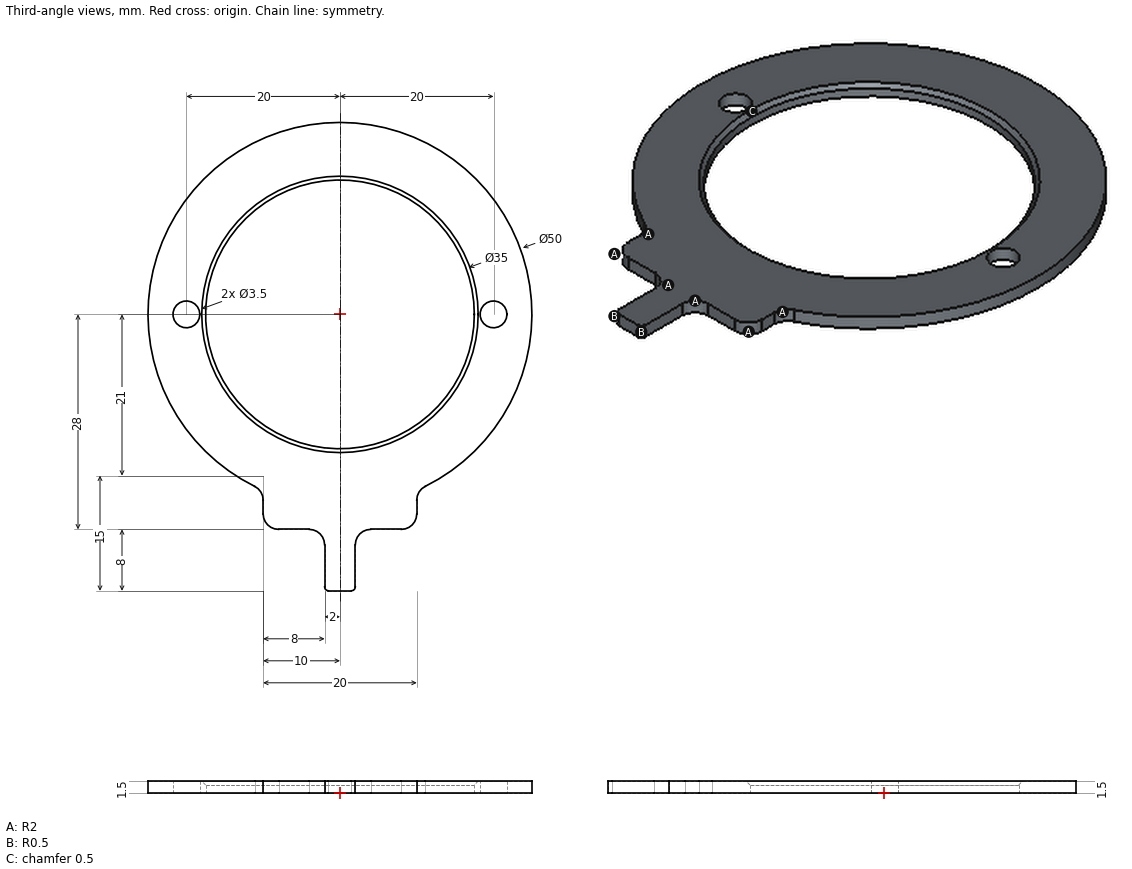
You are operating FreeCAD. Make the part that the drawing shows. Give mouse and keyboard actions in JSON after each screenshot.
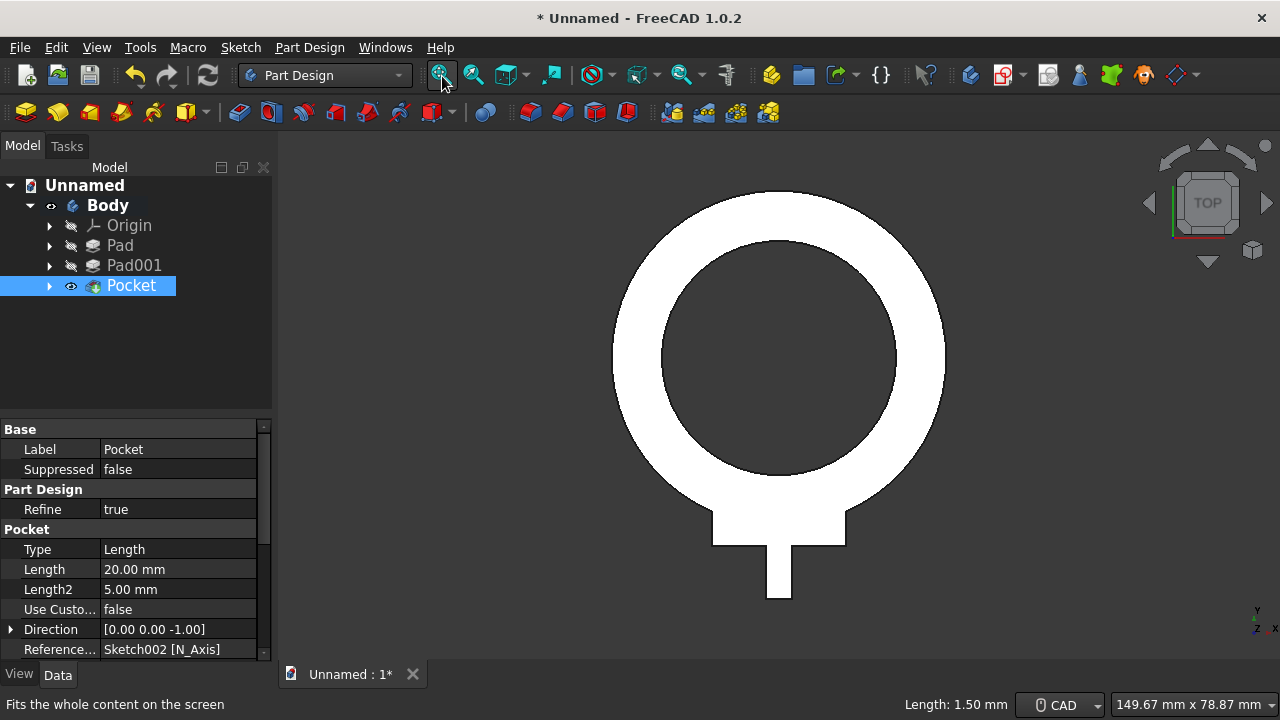
{"action": "scroll", "coordinate": [846, 511], "scroll_direction": "up", "scroll_amount": 7}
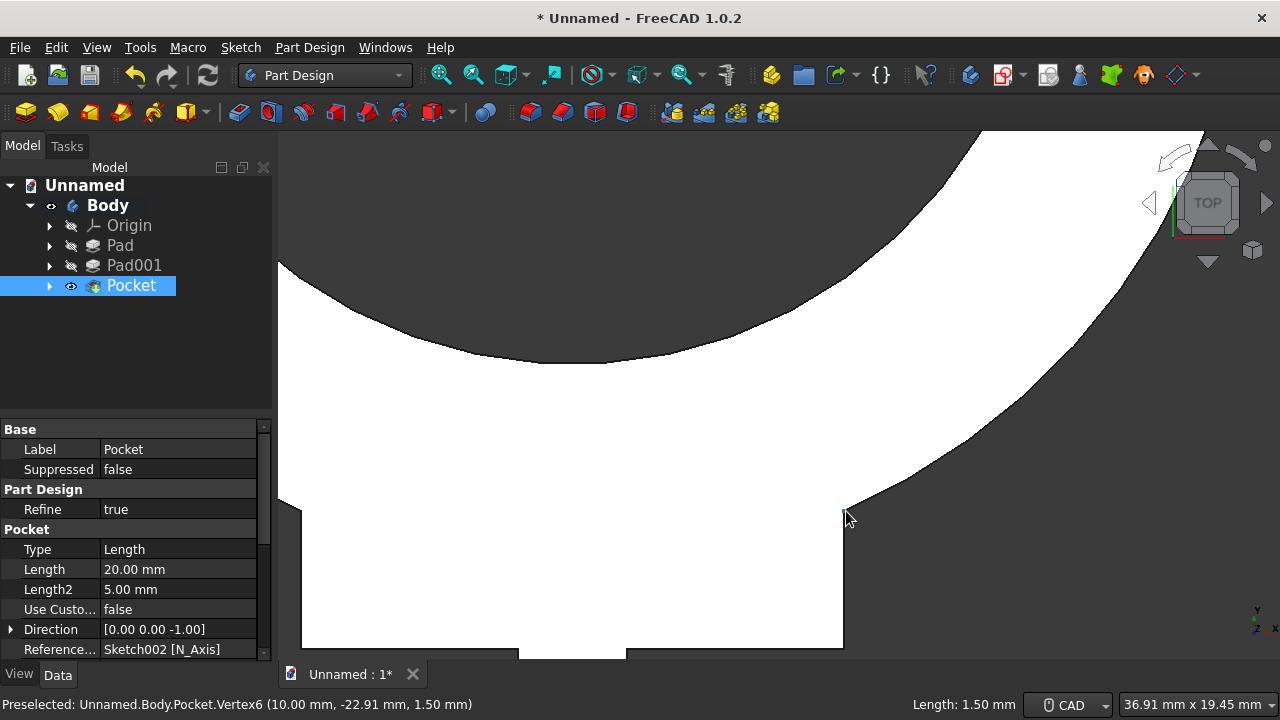
{"action": "left_click", "coordinate": [442, 76]}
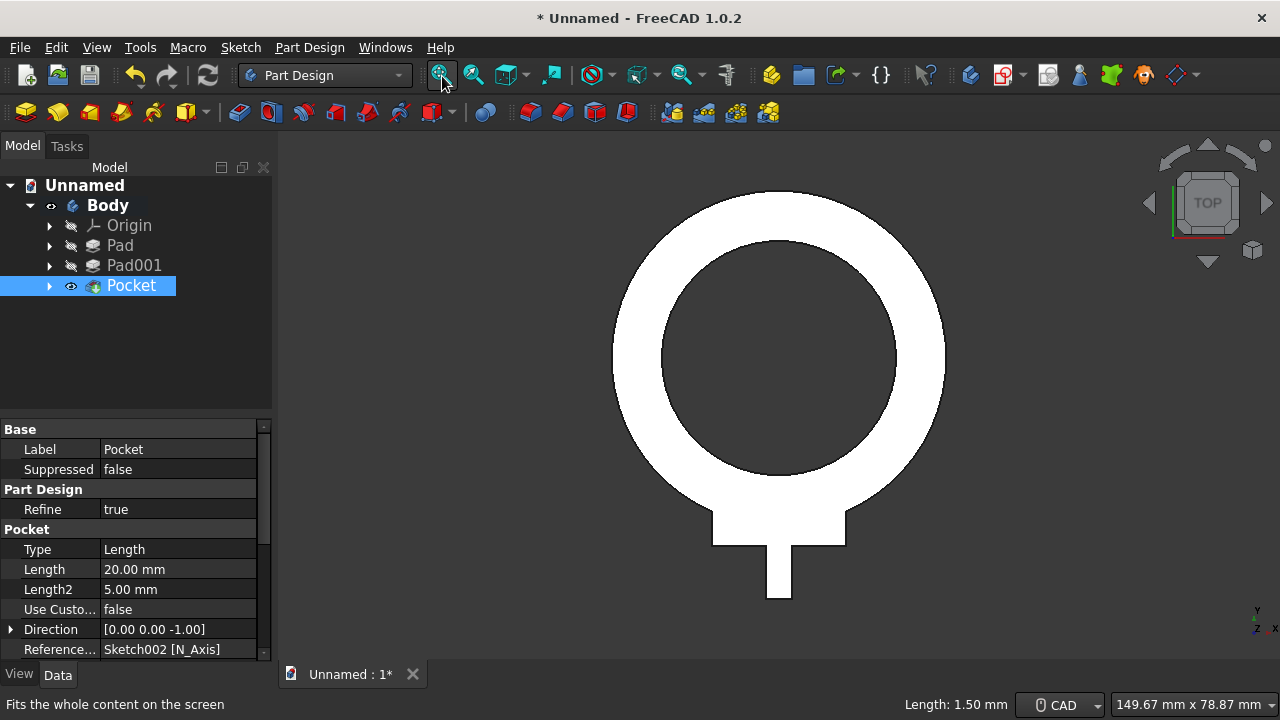
{"action": "key", "text": "1"}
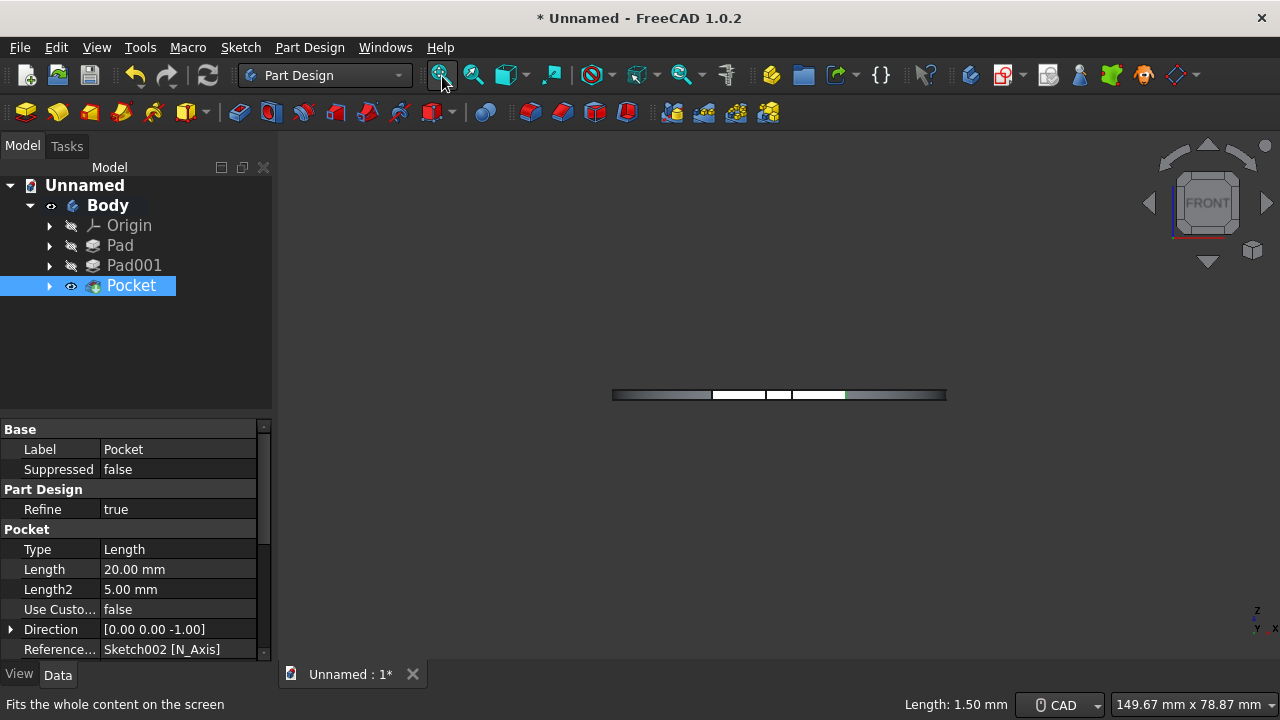
{"action": "left_click", "coordinate": [442, 76]}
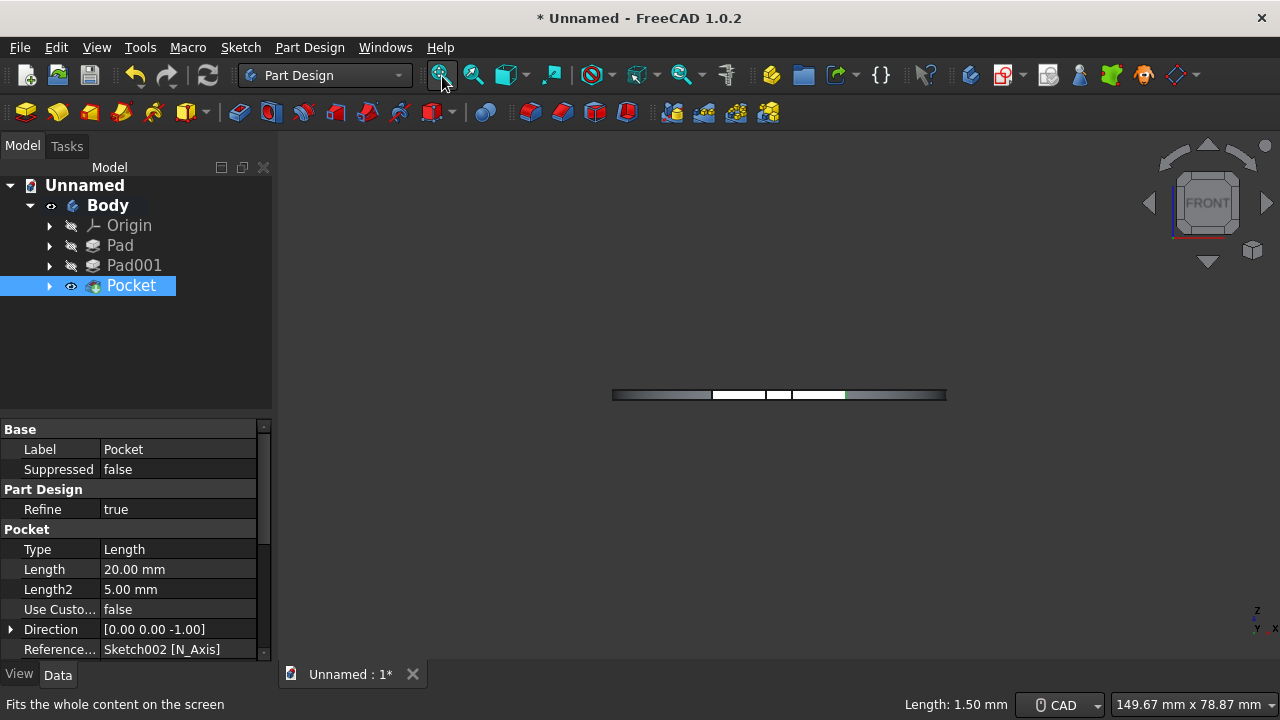
{"action": "scroll", "coordinate": [846, 394], "scroll_direction": "up", "scroll_amount": 7}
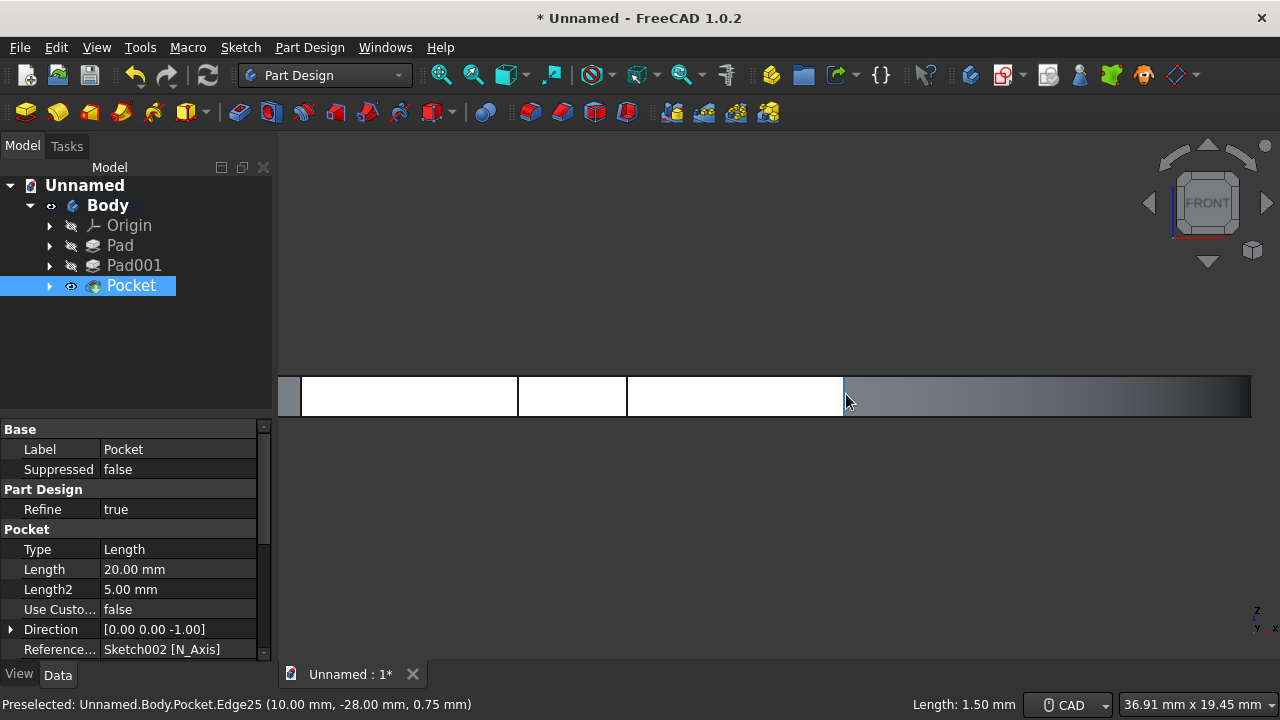
{"action": "left_click", "coordinate": [442, 76]}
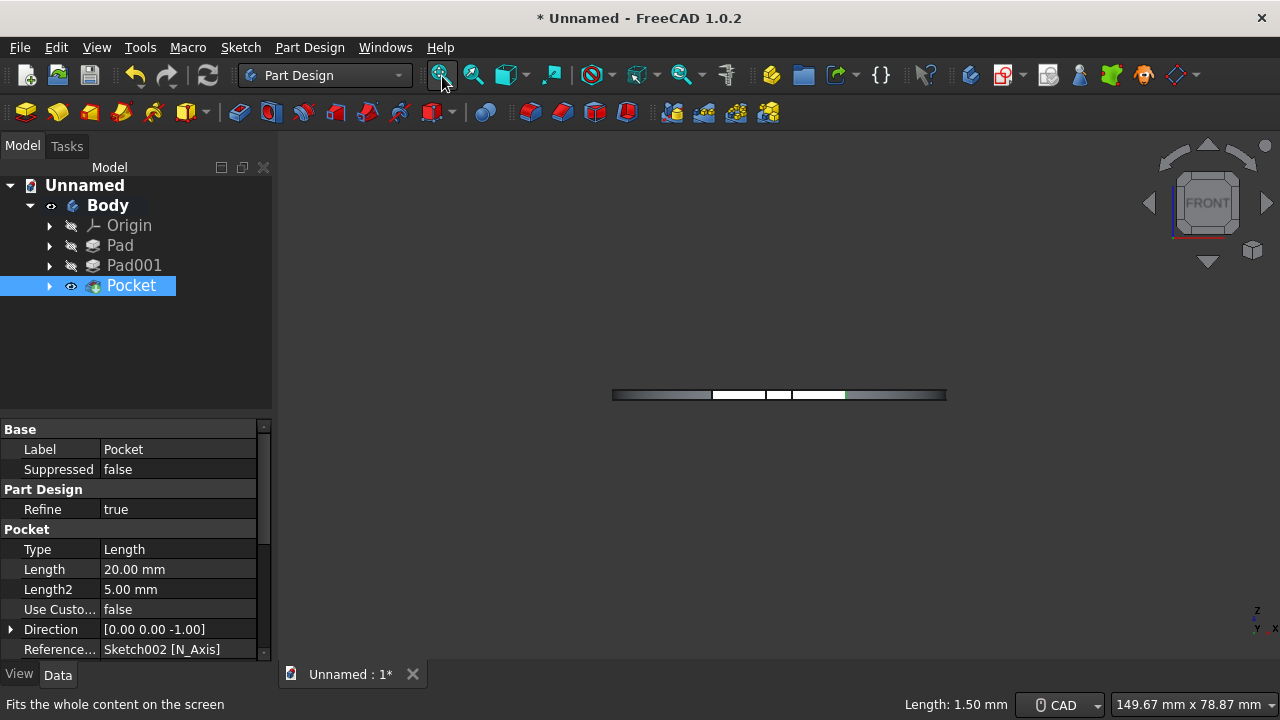
{"action": "key", "text": "3"}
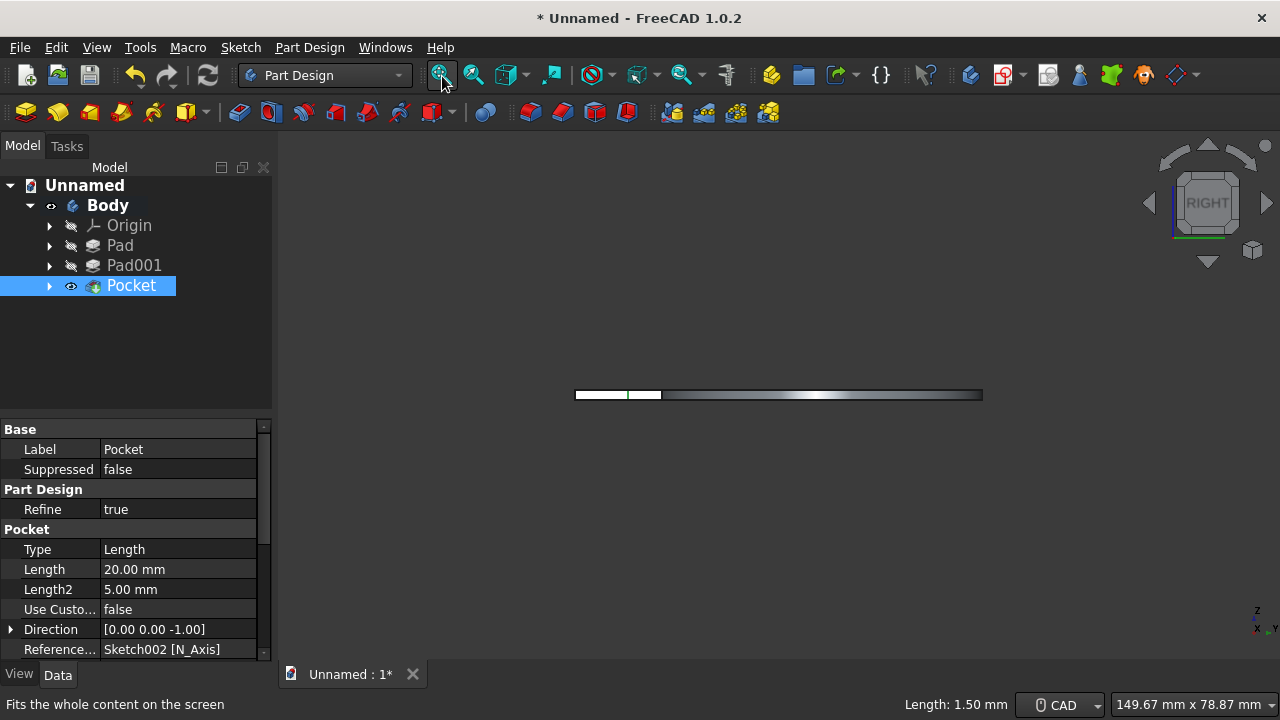
{"action": "left_click", "coordinate": [442, 76]}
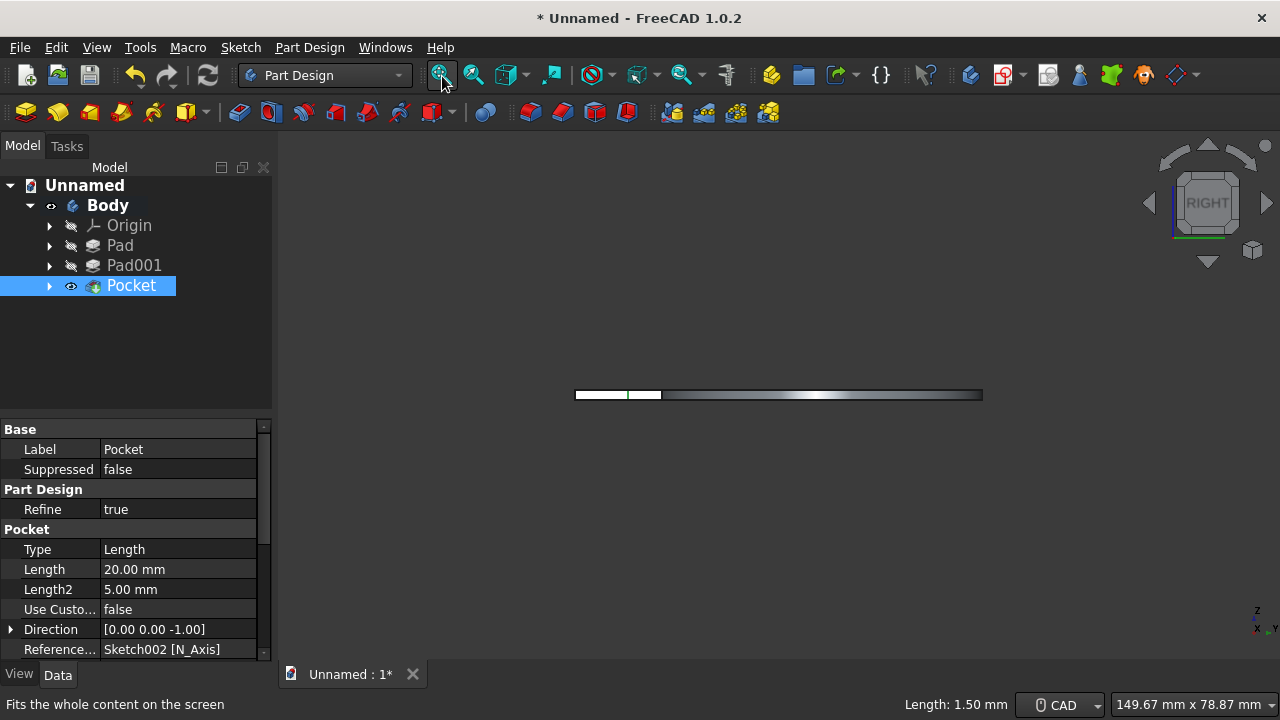
{"action": "scroll", "coordinate": [662, 394], "scroll_direction": "up", "scroll_amount": 7}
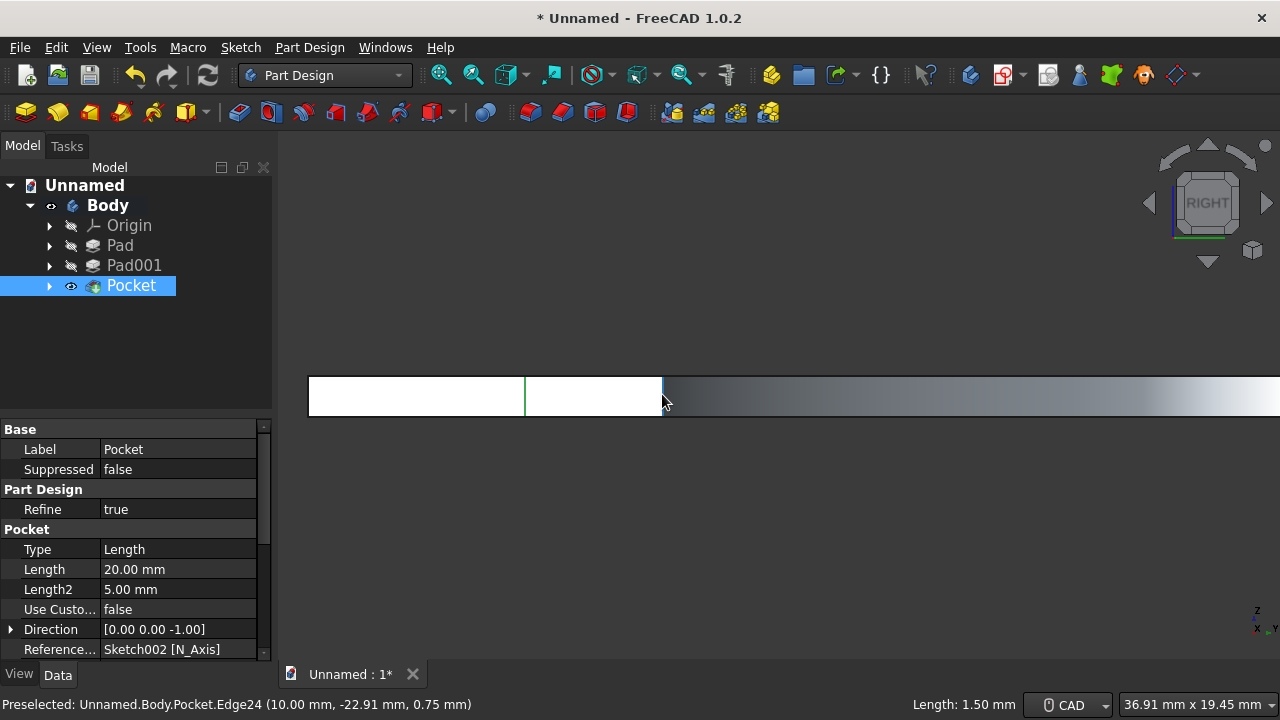
{"action": "left_click", "coordinate": [442, 76]}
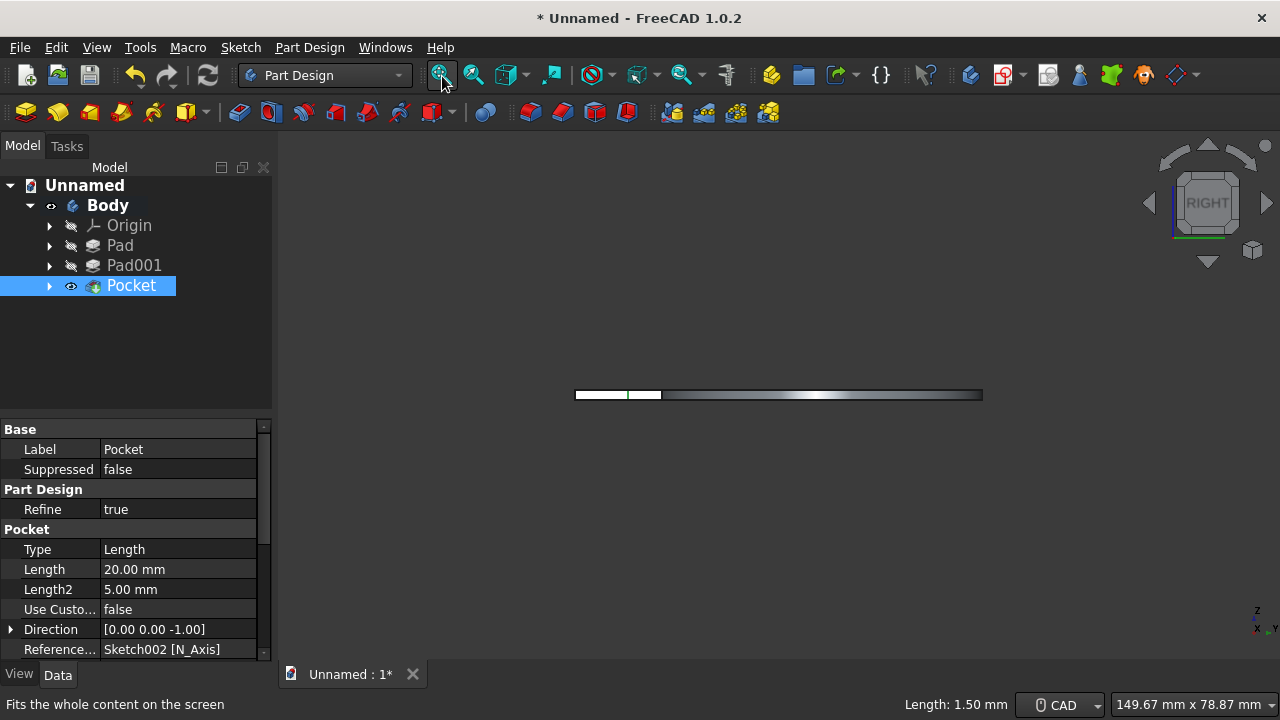
{"action": "key", "text": "5"}